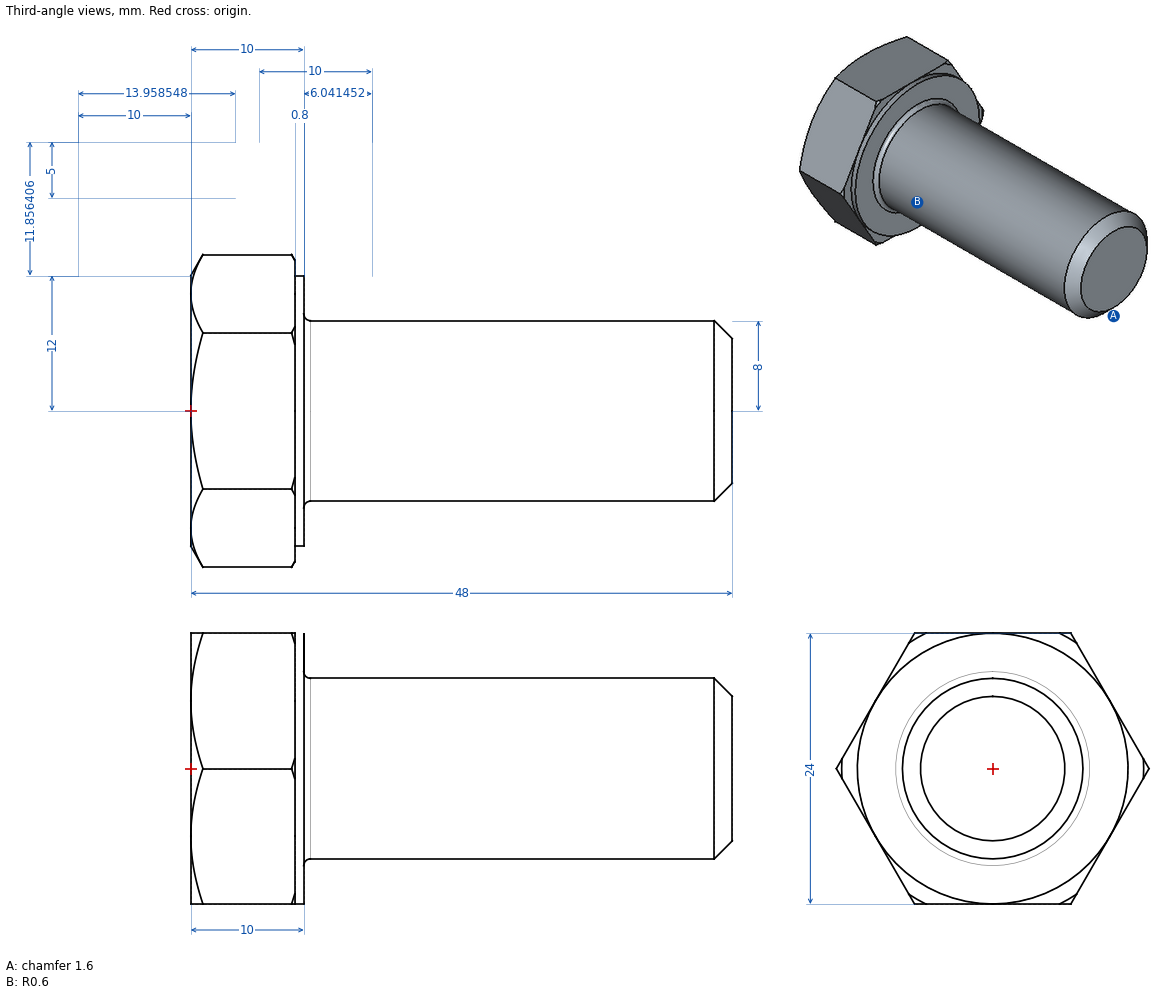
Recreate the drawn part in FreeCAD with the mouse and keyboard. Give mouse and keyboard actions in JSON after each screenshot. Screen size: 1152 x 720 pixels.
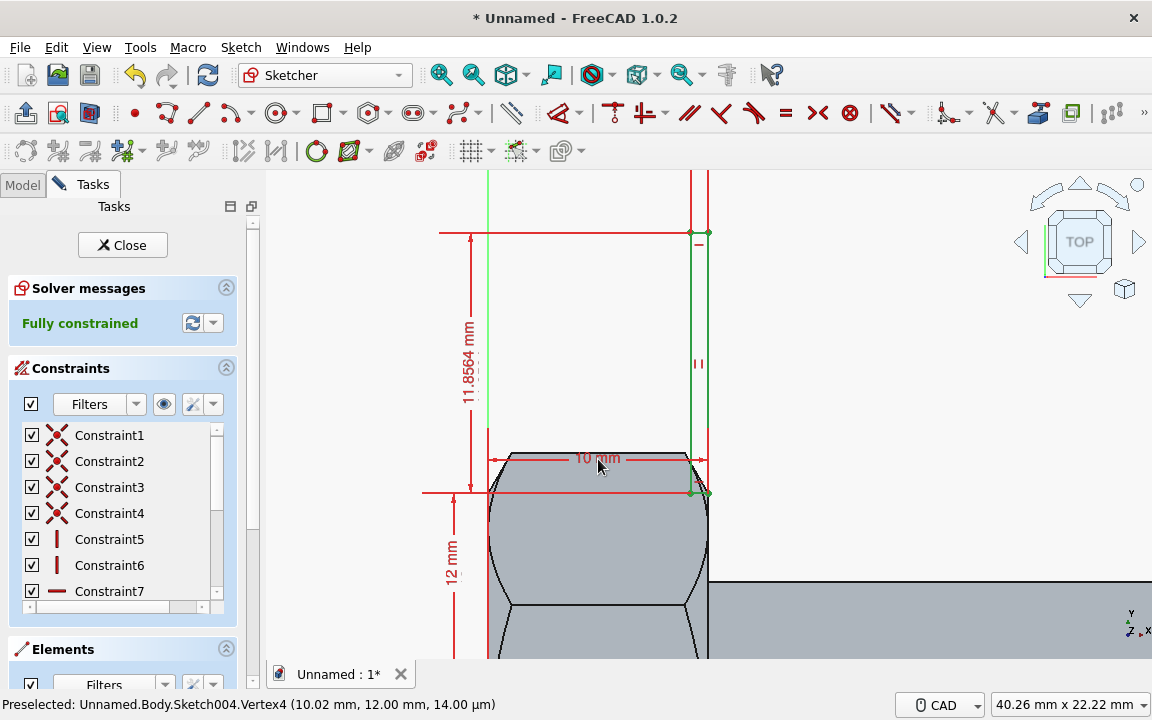
{"action": "left_click", "coordinate": [123, 245]}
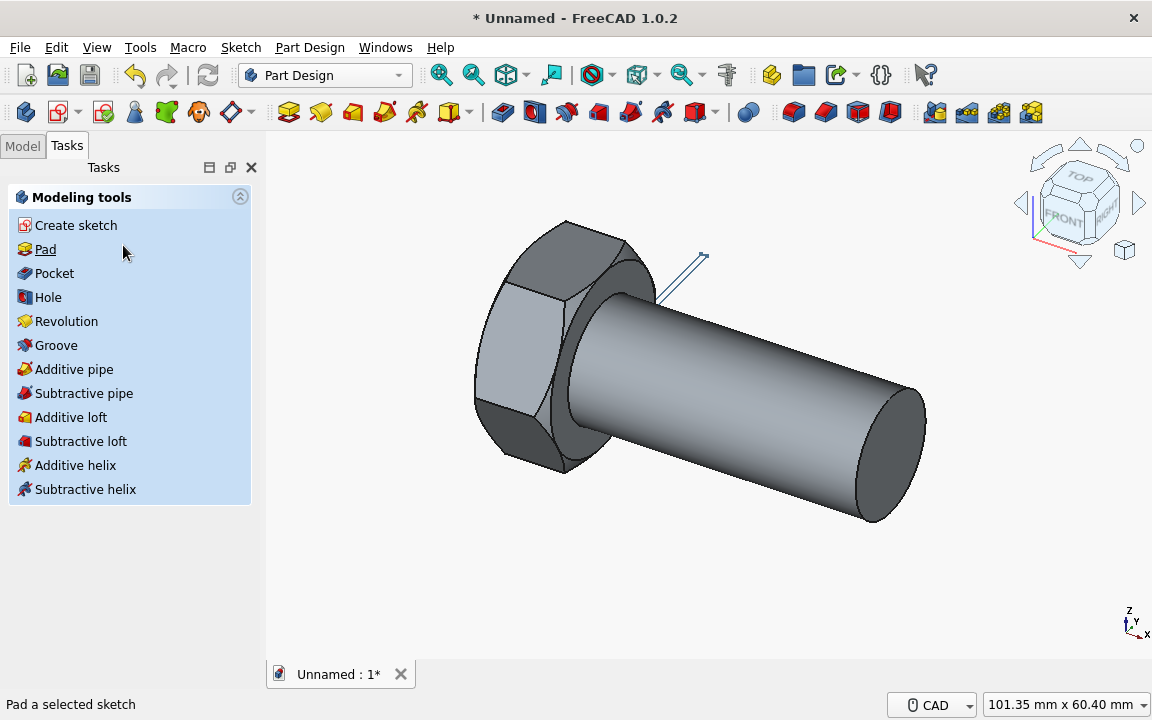
{"action": "left_click", "coordinate": [568, 112]}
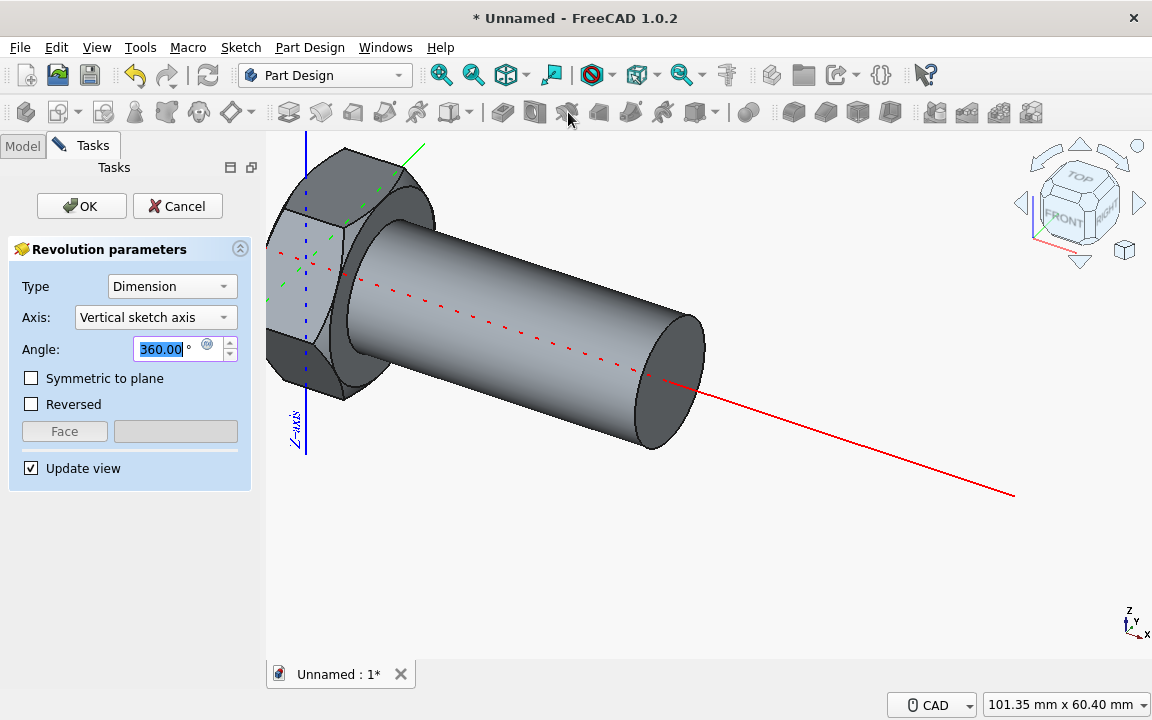
{"action": "left_click", "coordinate": [156, 318]}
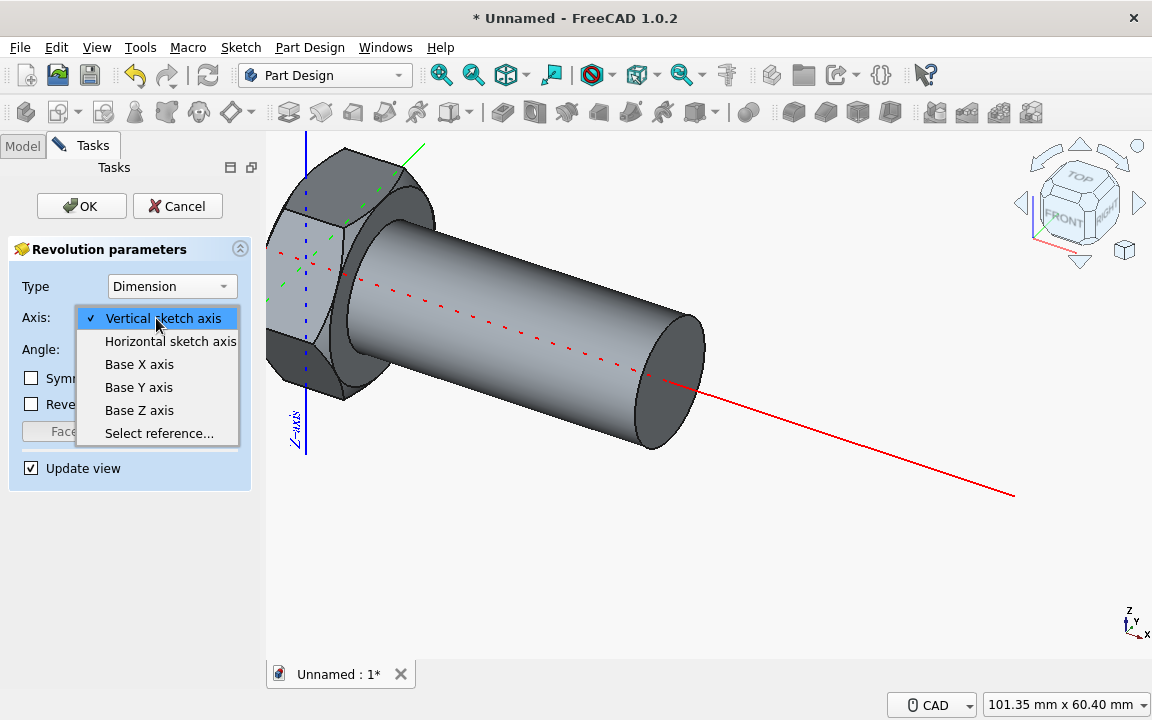
{"action": "left_click", "coordinate": [156, 342]}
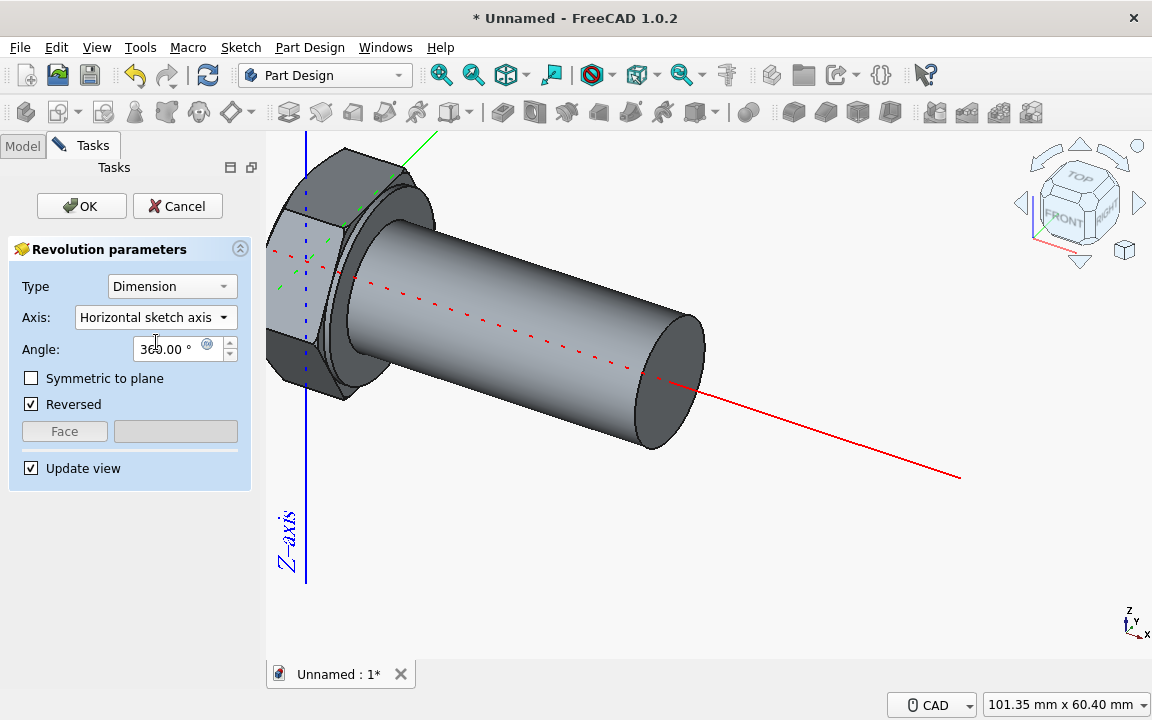
{"action": "left_click", "coordinate": [82, 206]}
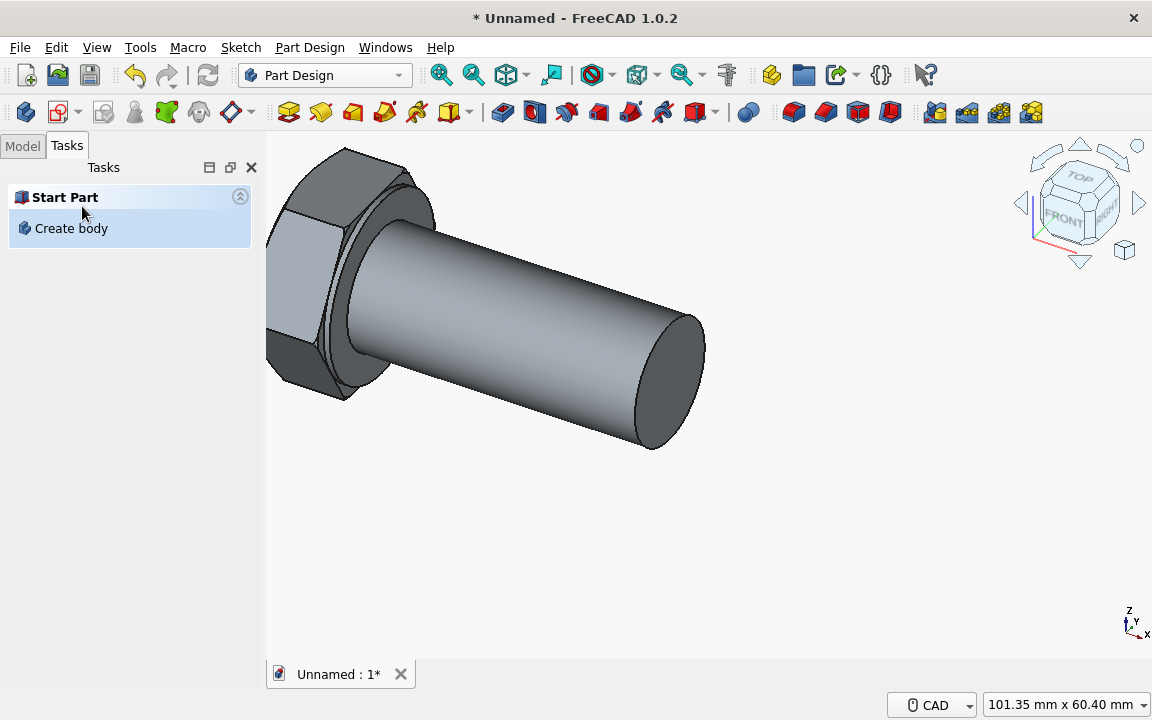
{"action": "left_click", "coordinate": [442, 76]}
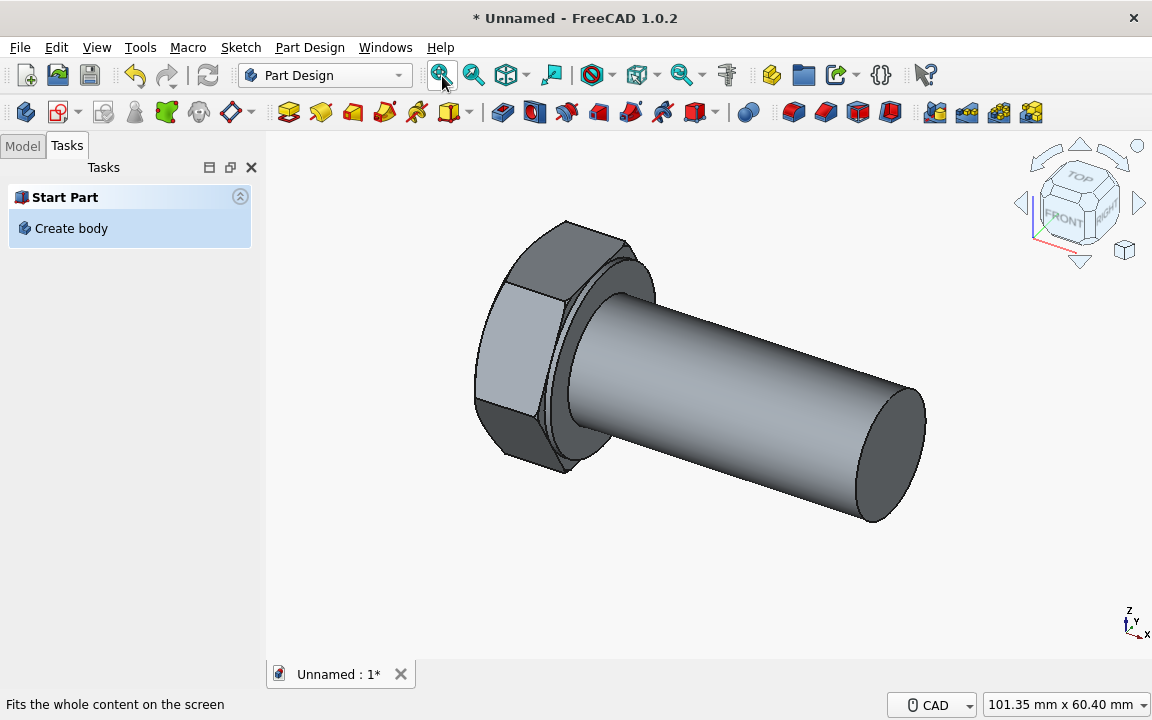
{"action": "left_click", "coordinate": [856, 489]}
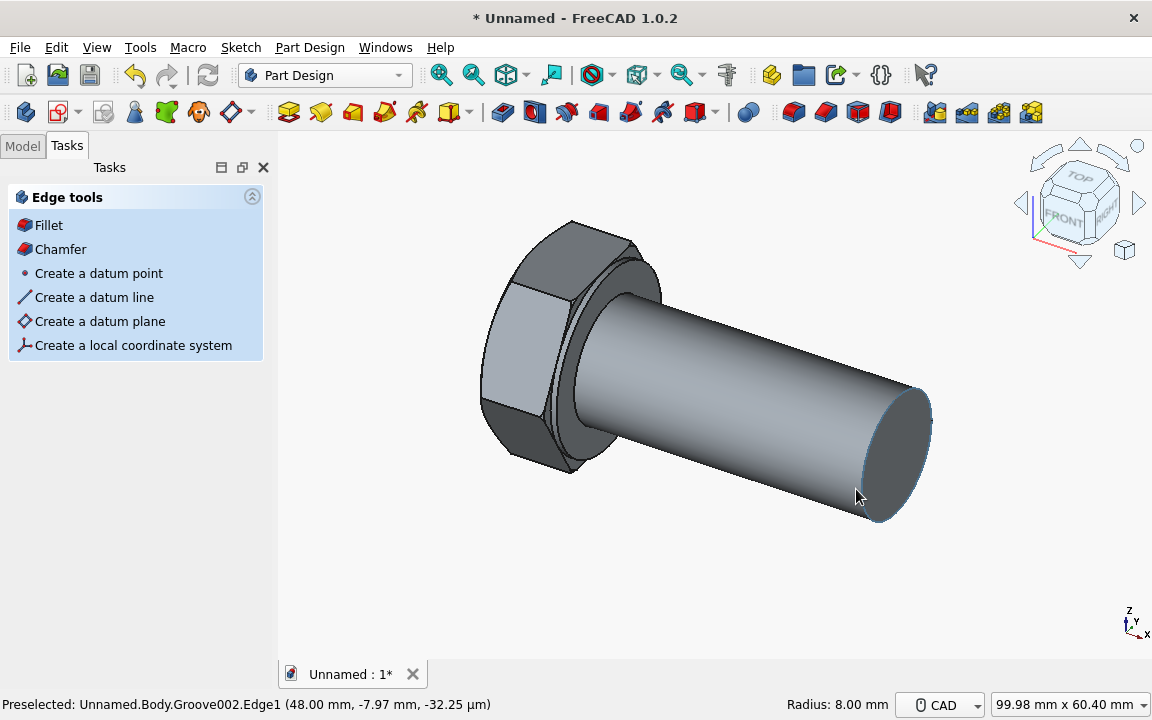
{"action": "left_click", "coordinate": [826, 112]}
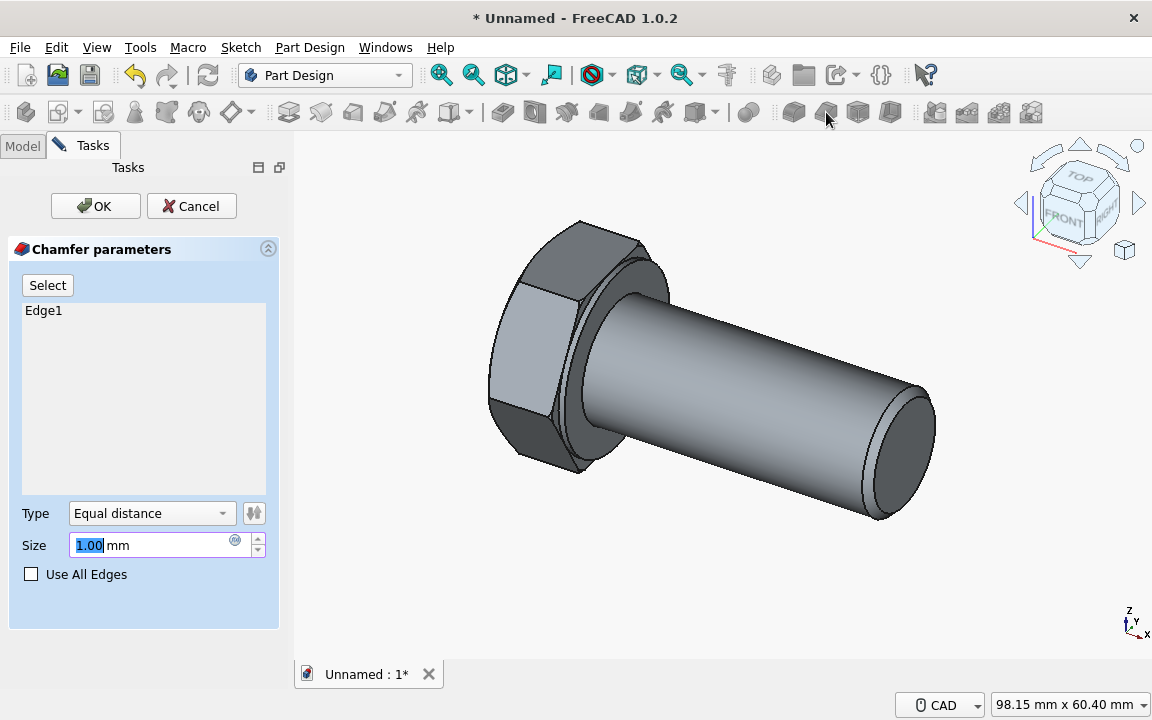
{"action": "type", "text": "1.6"}
{"action": "key", "text": "Tab"}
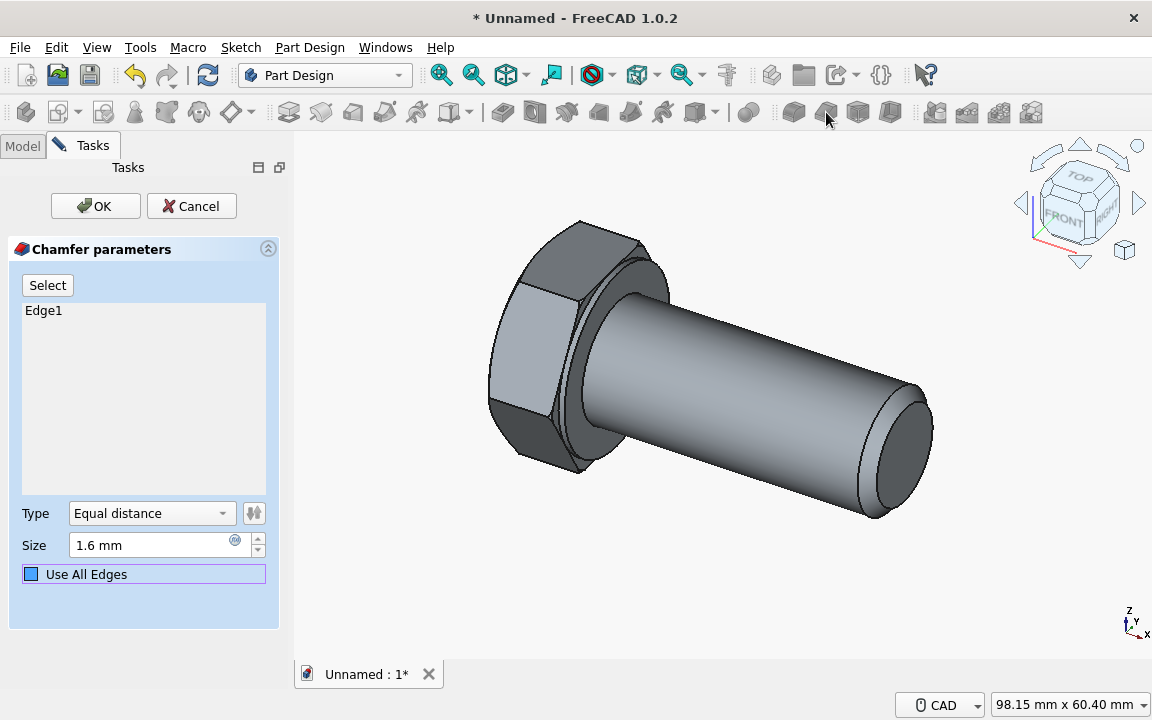
{"action": "left_click", "coordinate": [96, 206]}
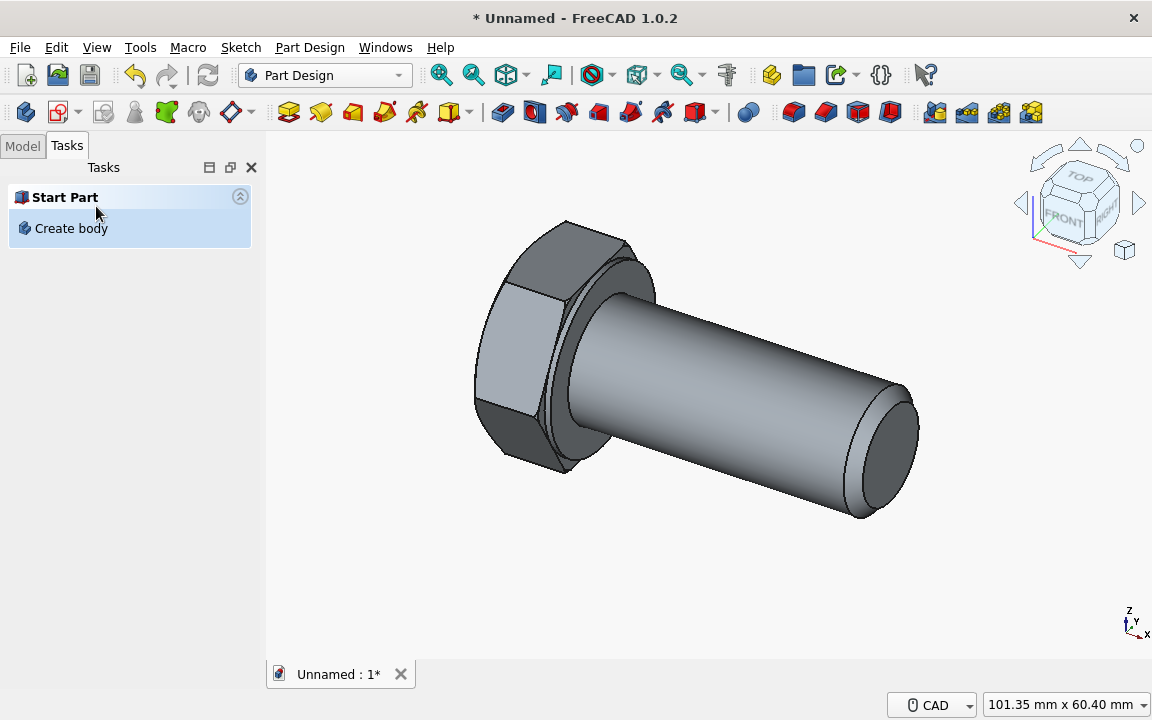
{"action": "key", "text": "0"}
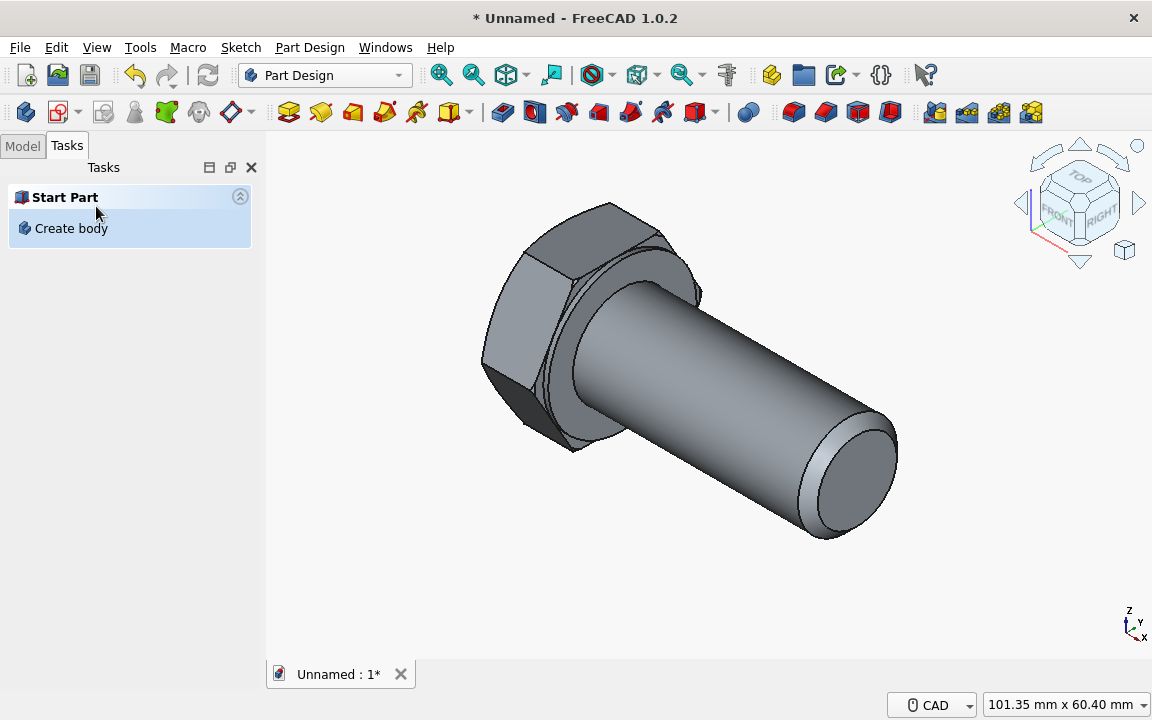
{"action": "key", "text": "2"}